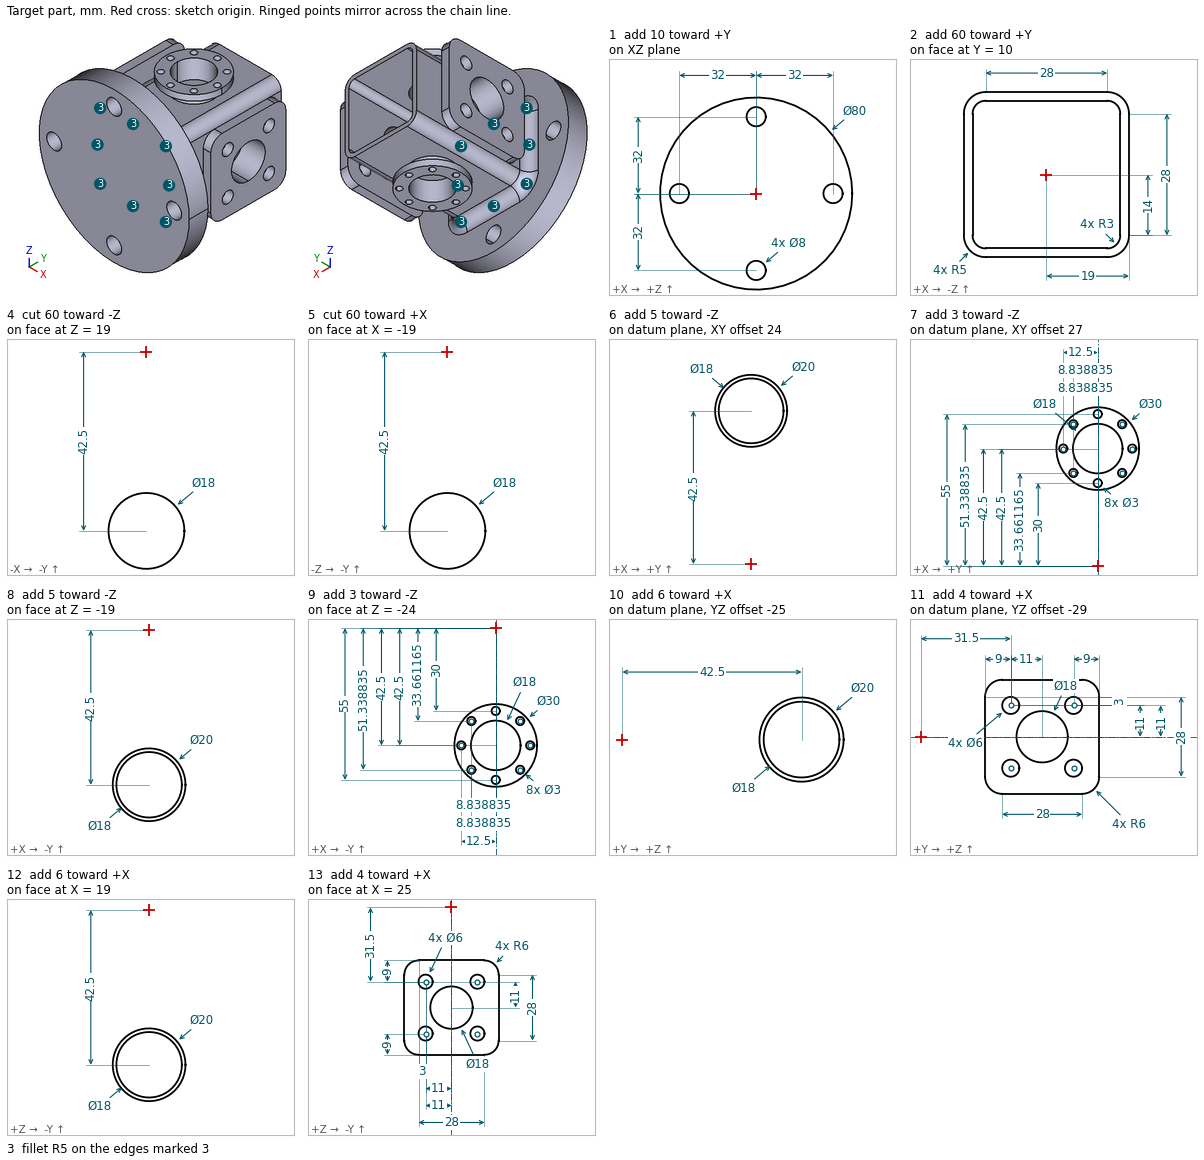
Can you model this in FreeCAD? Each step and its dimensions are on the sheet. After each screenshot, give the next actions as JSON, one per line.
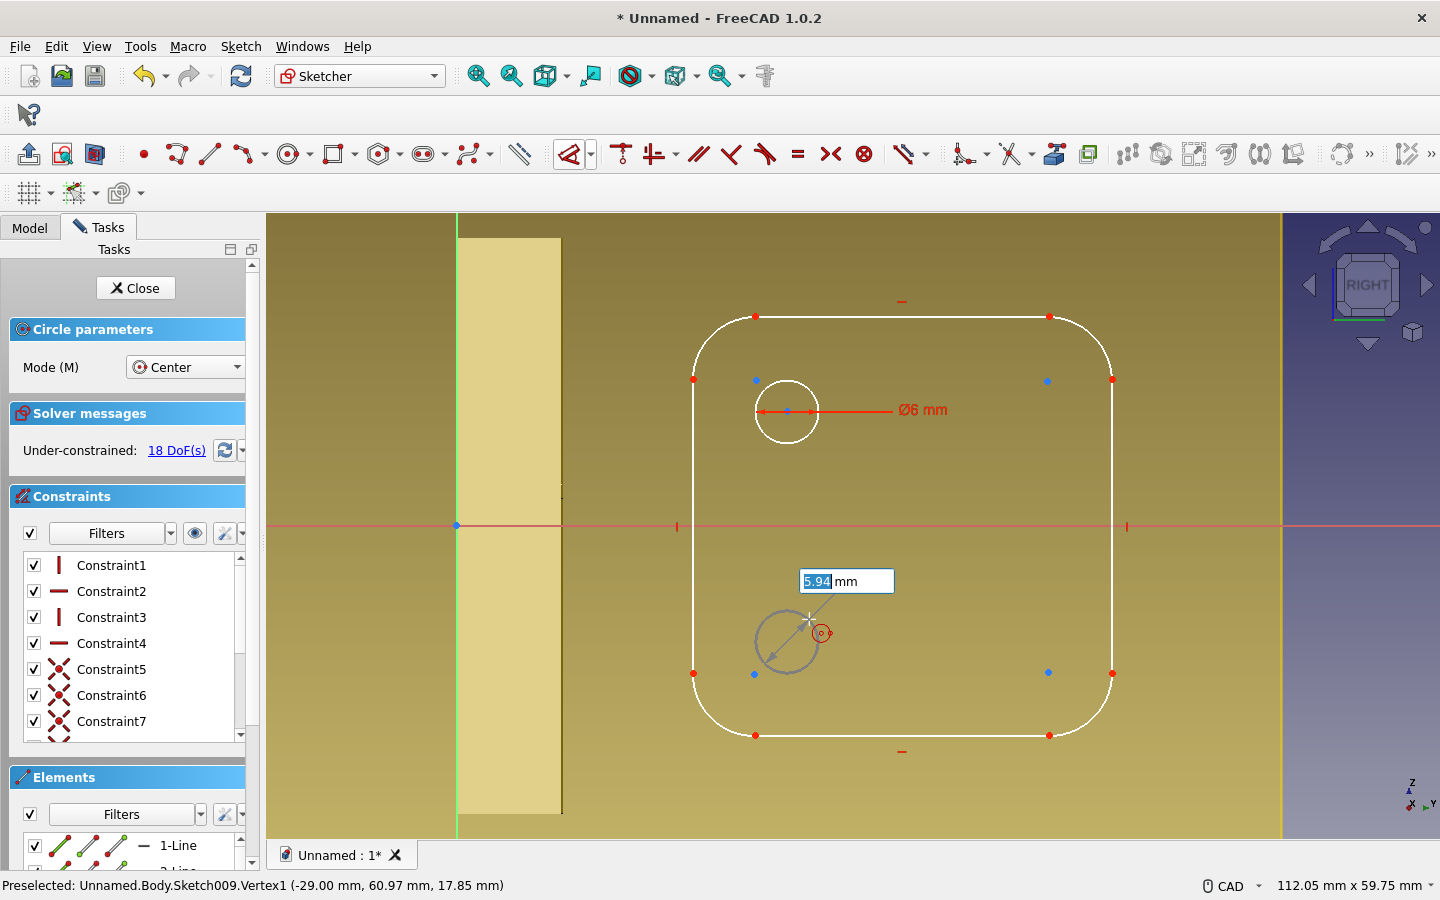
{"action": "type", "text": "6"}
{"action": "key", "text": "Return"}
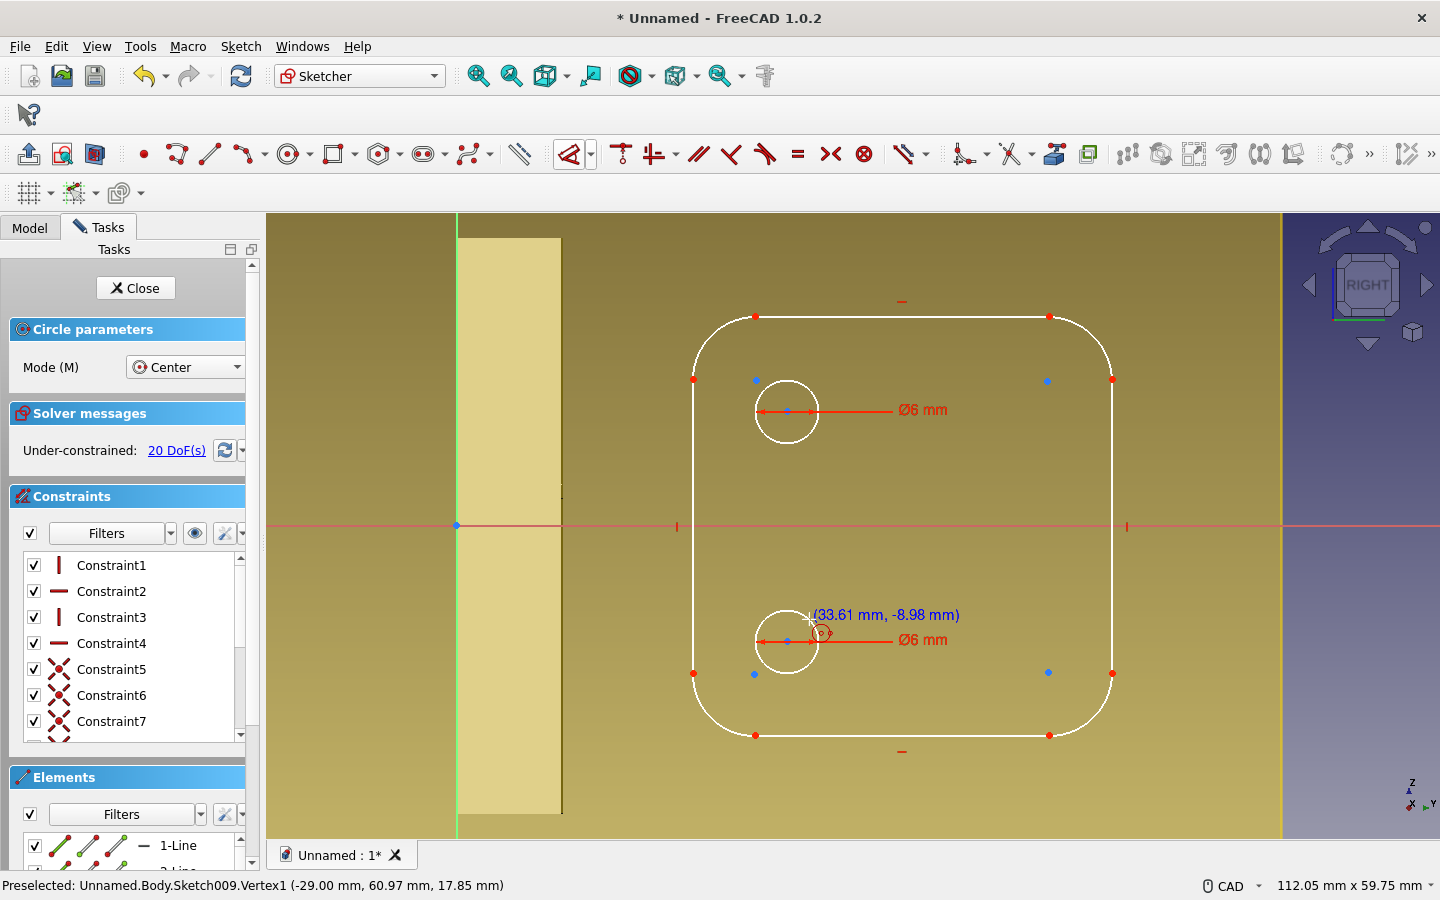
{"action": "left_click", "coordinate": [1017, 411]}
{"action": "mouse_move", "coordinate": [995, 388]}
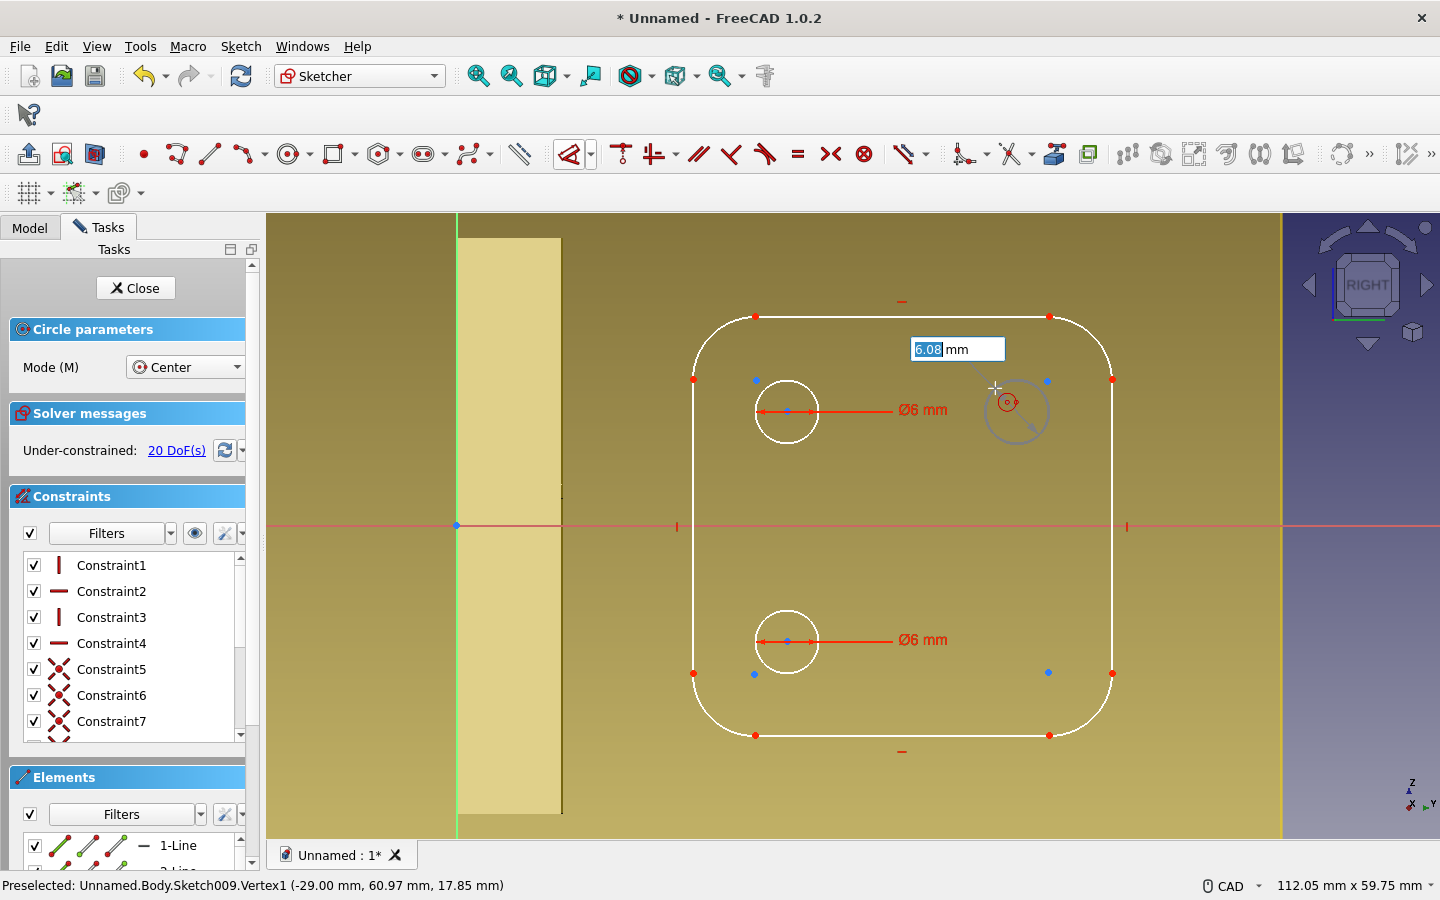
{"action": "type", "text": "6"}
{"action": "key", "text": "Return"}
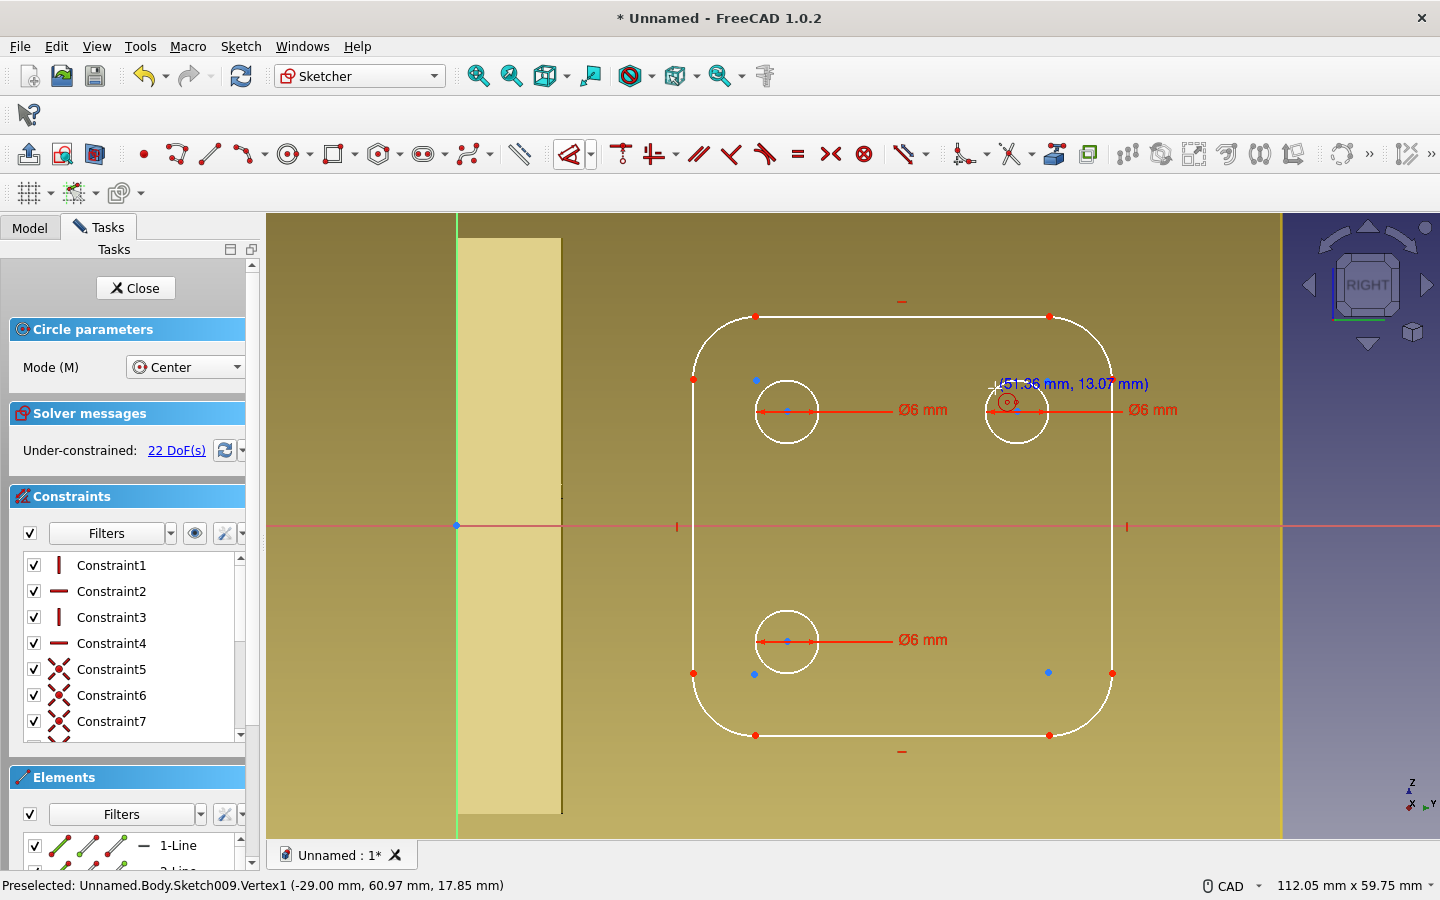
{"action": "left_click", "coordinate": [902, 526]}
{"action": "mouse_move", "coordinate": [969, 459]}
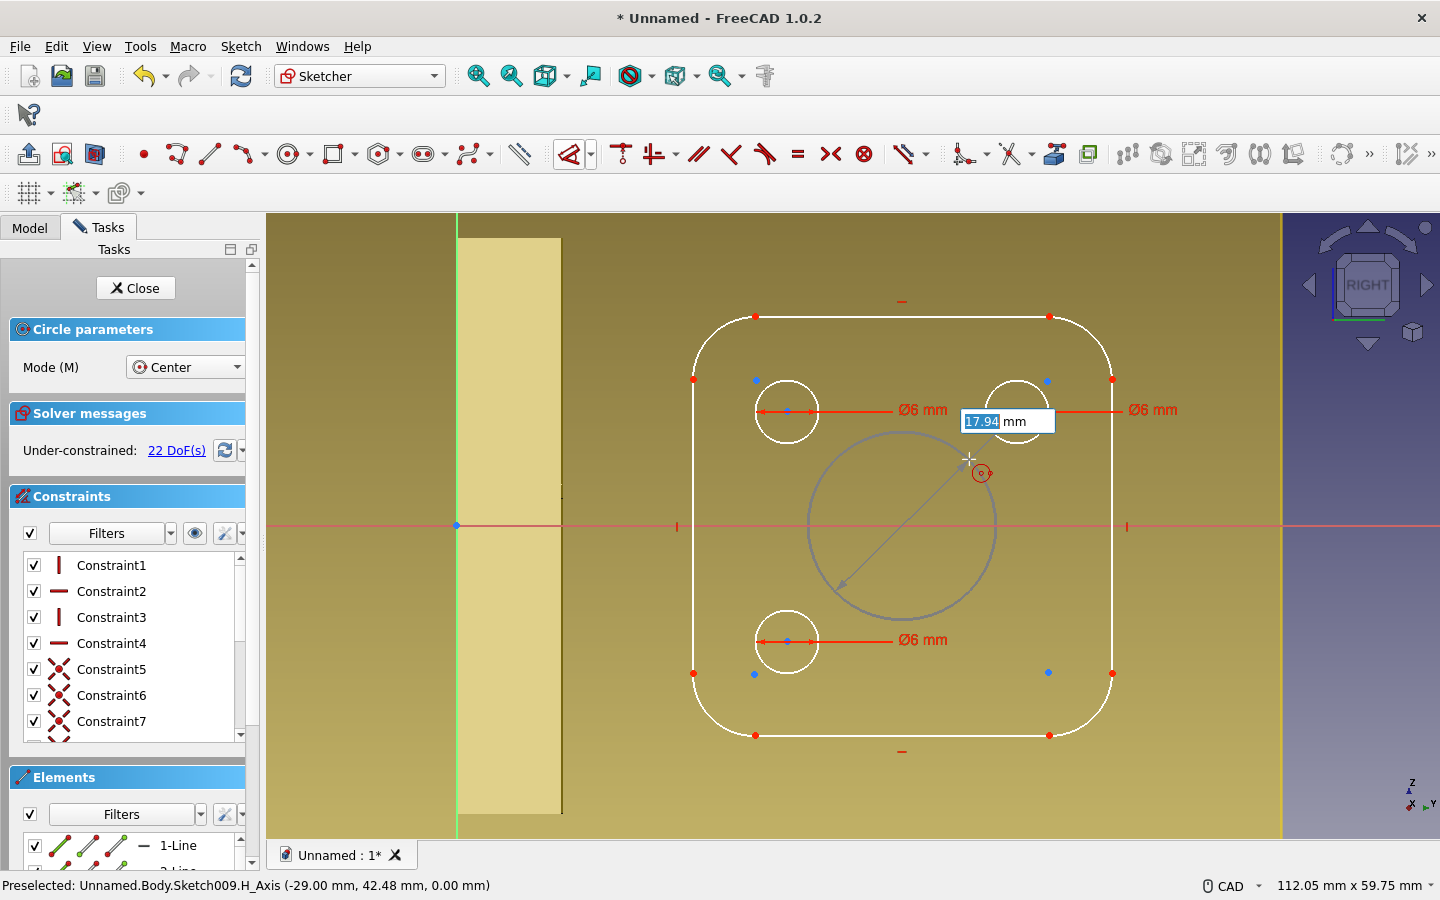
{"action": "type", "text": "18"}
{"action": "key", "text": "Return"}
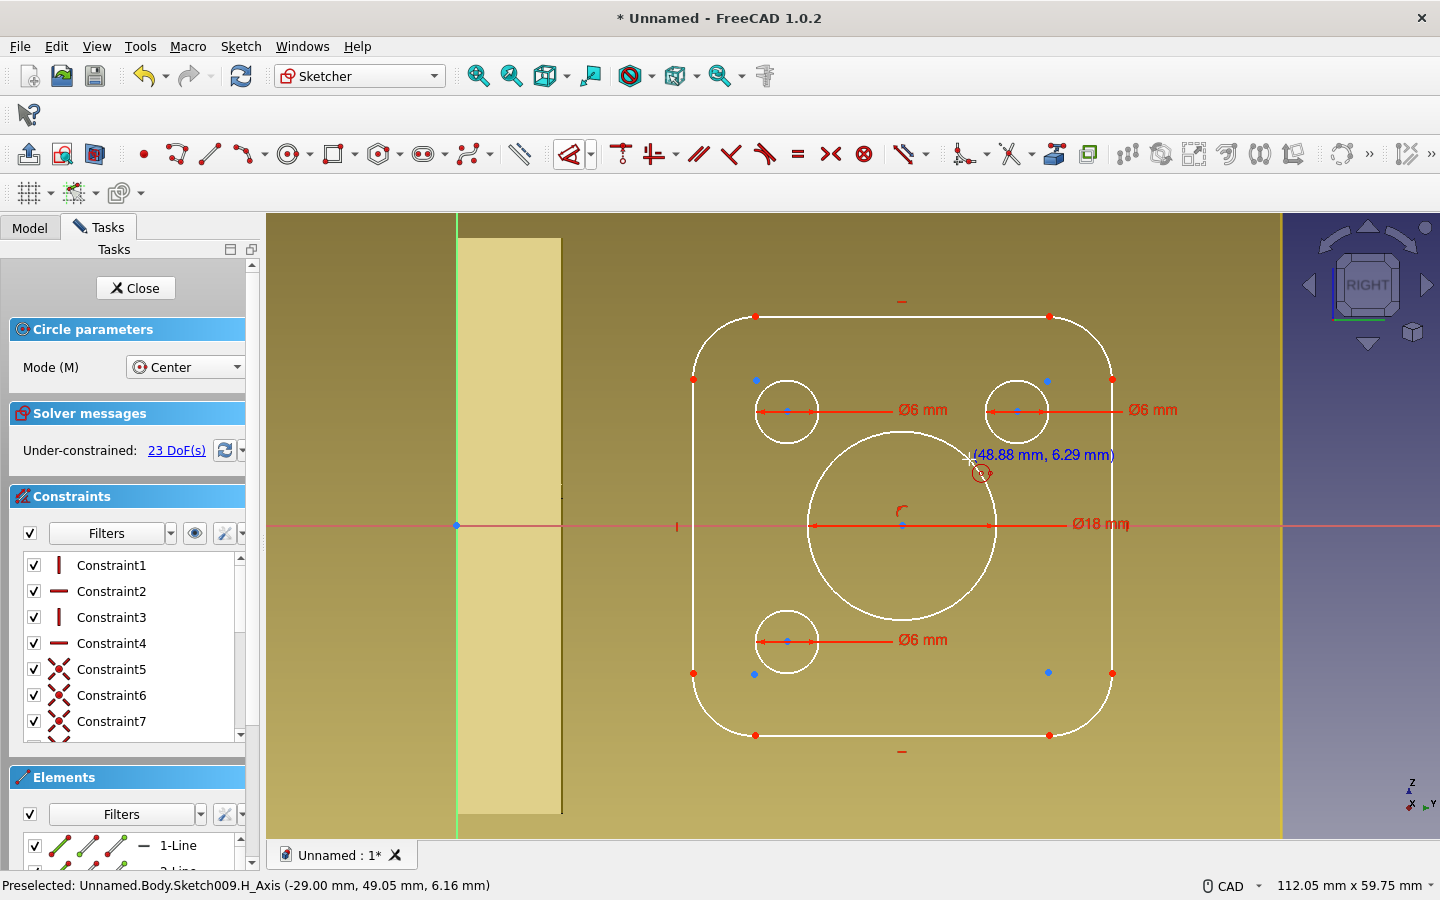
{"action": "left_click", "coordinate": [1017, 641]}
{"action": "mouse_move", "coordinate": [1040, 619]}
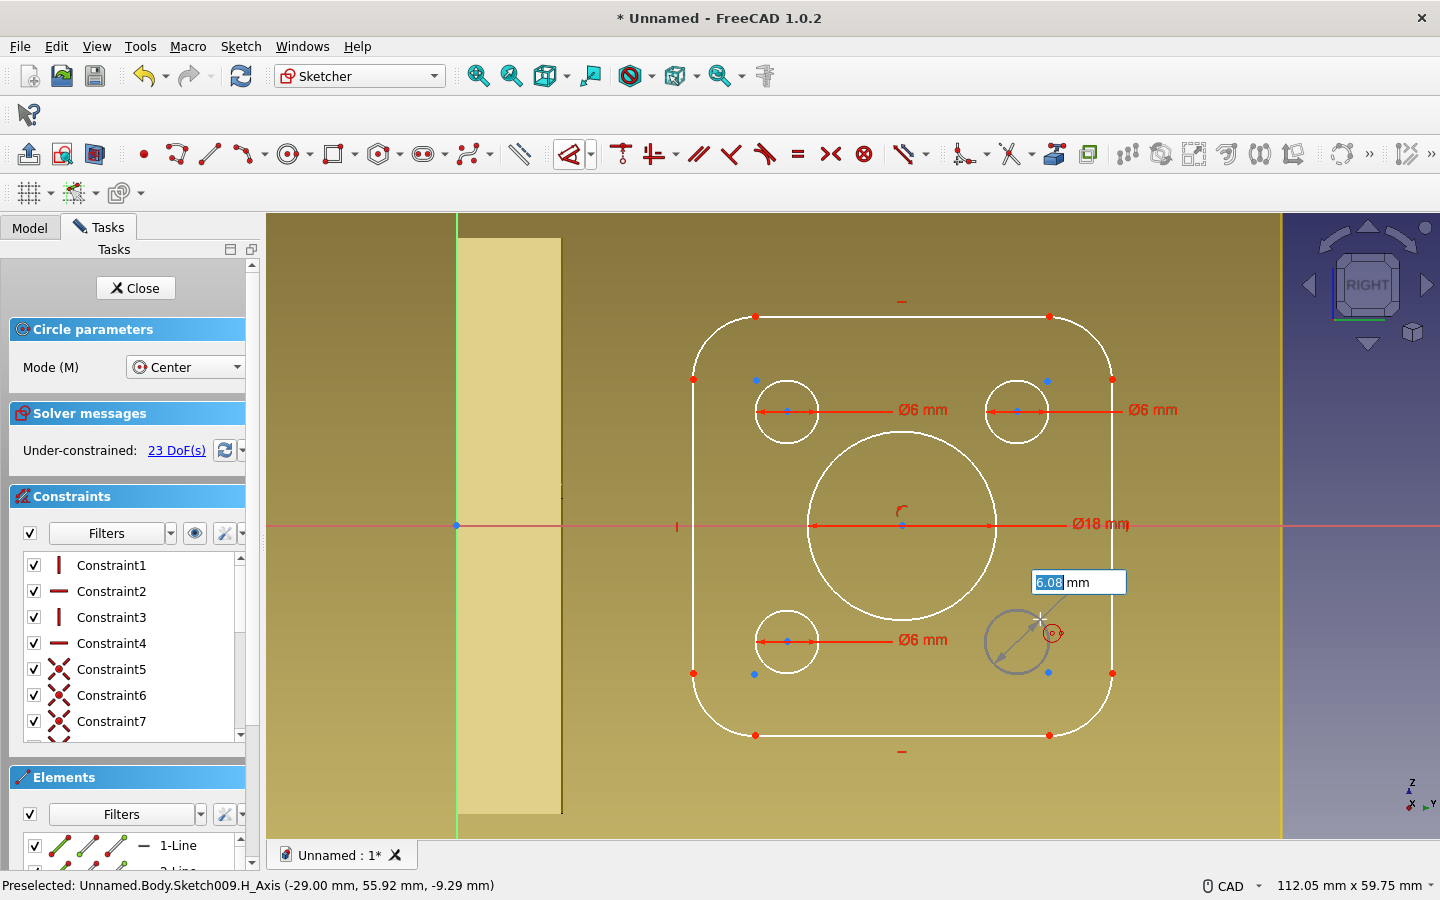
{"action": "type", "text": "6"}
{"action": "key", "text": "Return"}
{"action": "key", "text": "Escape"}